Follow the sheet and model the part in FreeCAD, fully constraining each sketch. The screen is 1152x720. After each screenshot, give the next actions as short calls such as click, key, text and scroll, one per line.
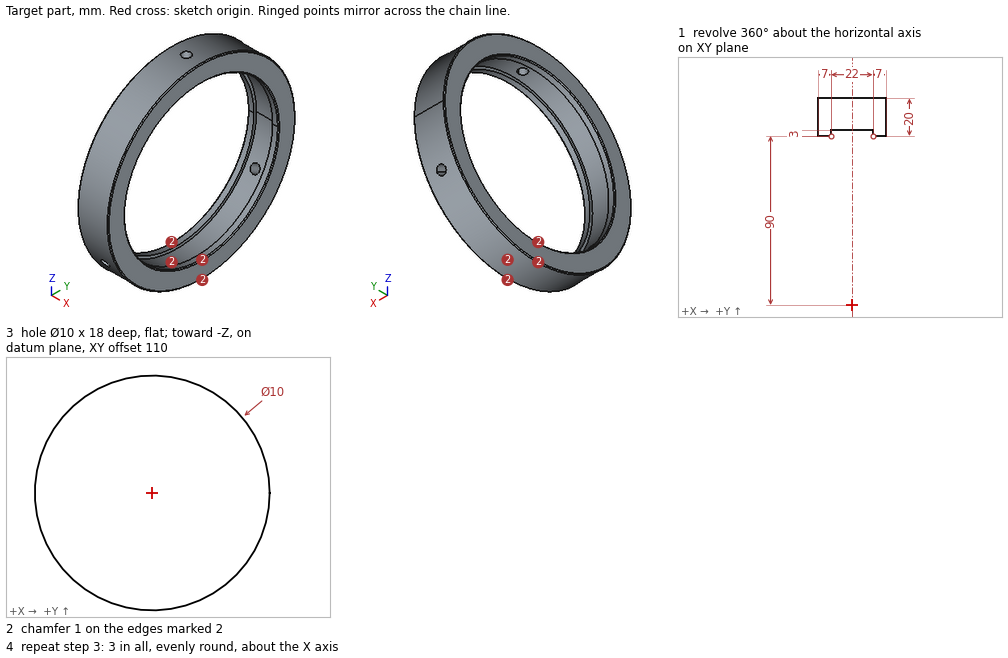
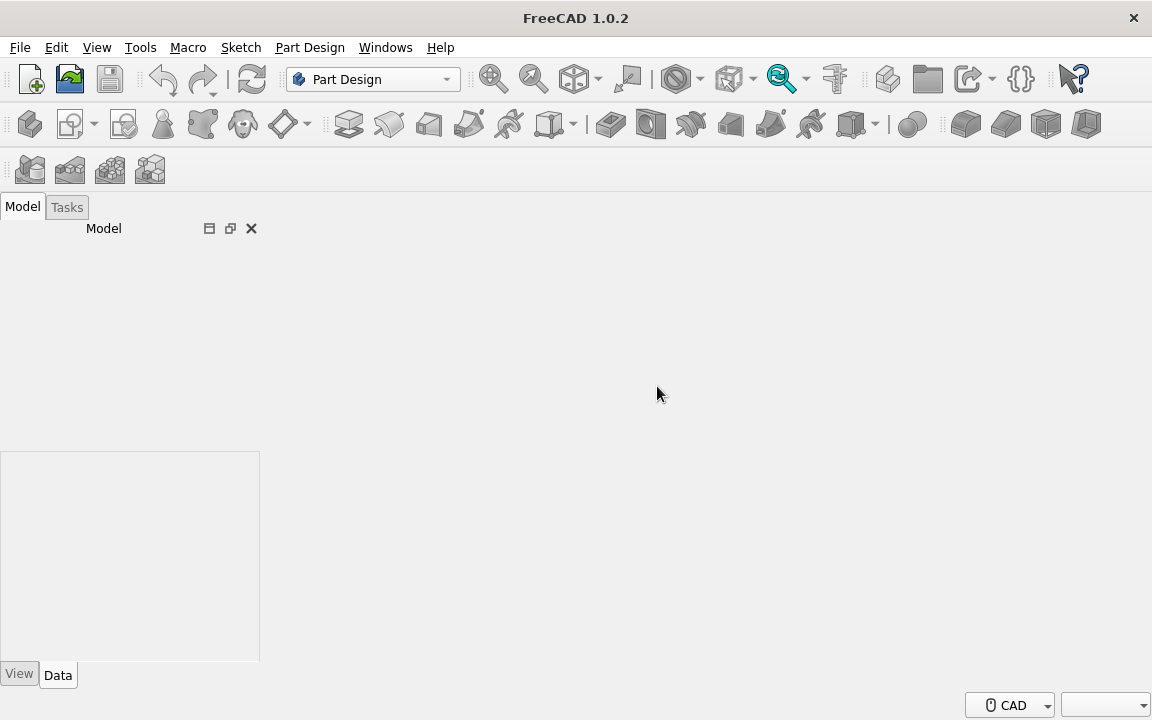
click(30, 80)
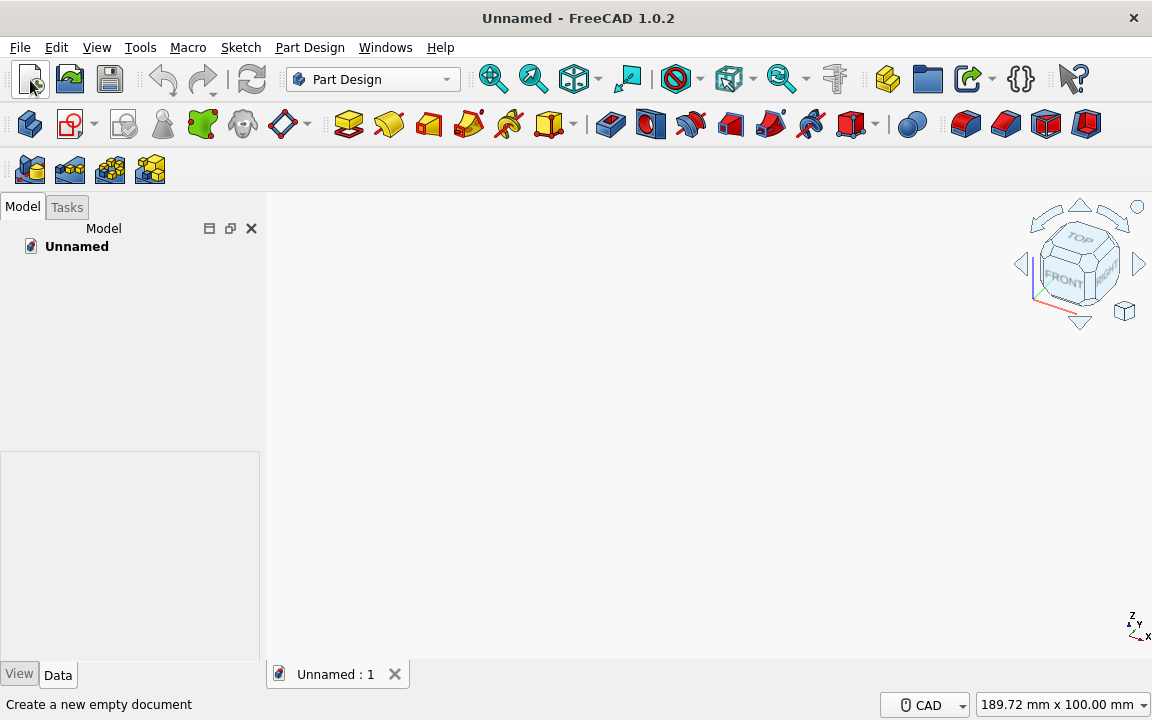
click(70, 124)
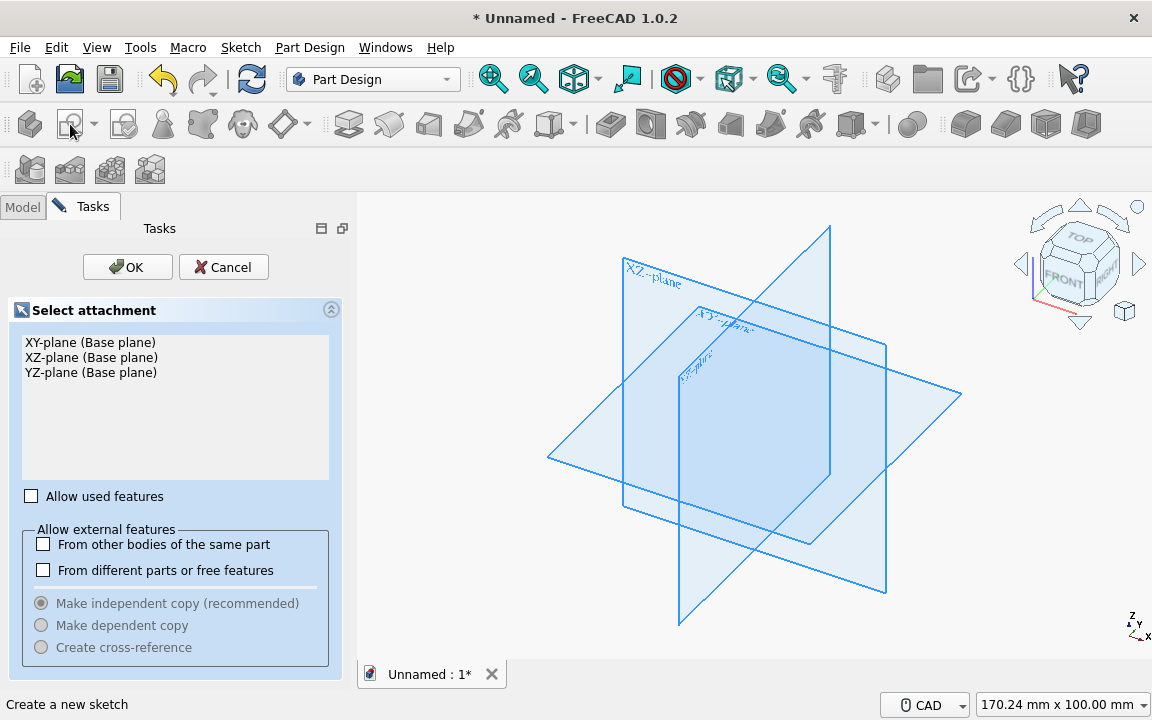
click(82, 342)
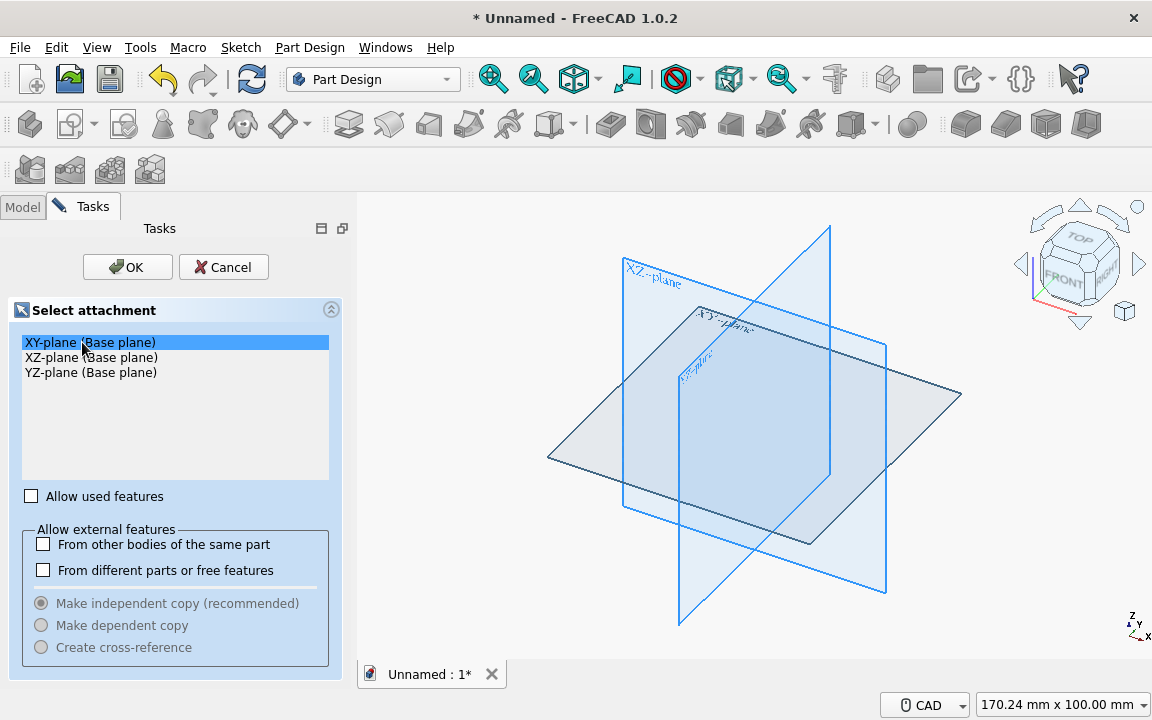
click(128, 267)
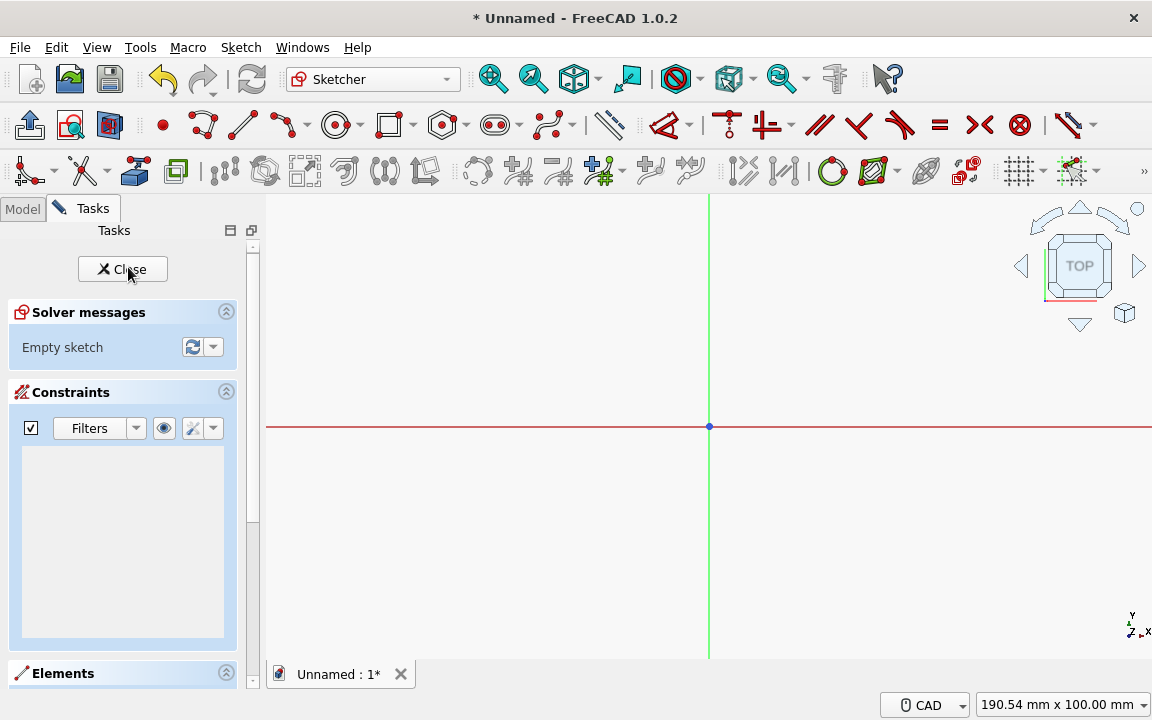
scroll(640, 426, down, 5)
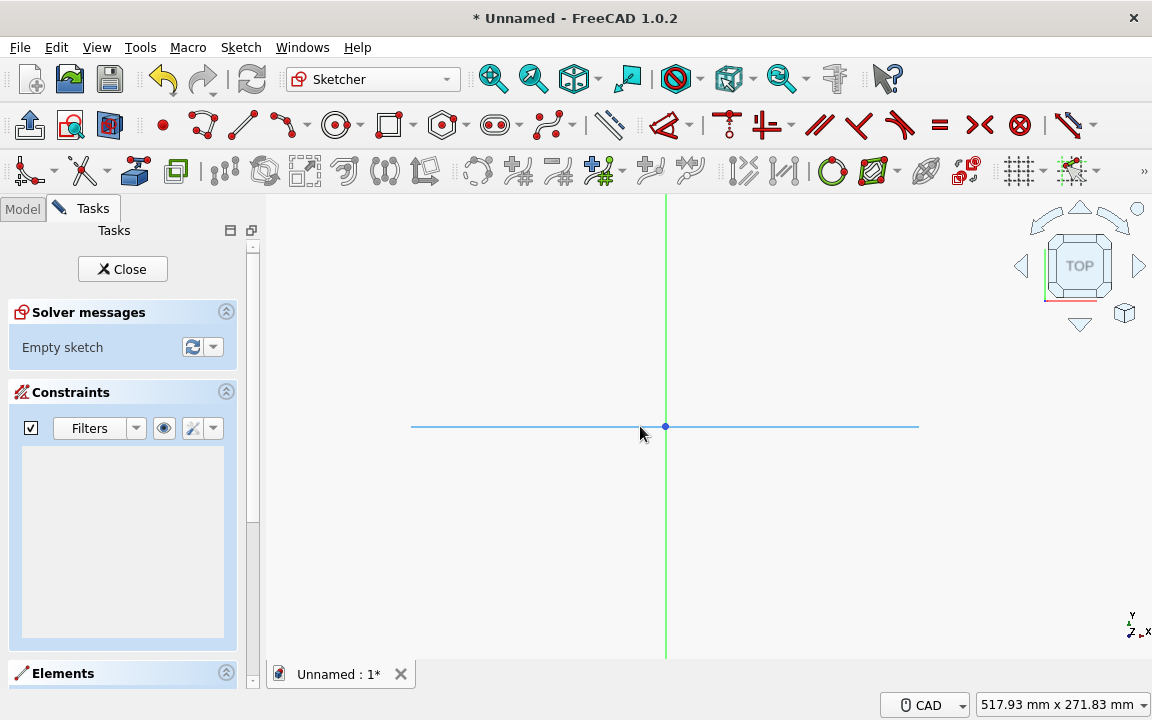
scroll(670, 229, up, 10)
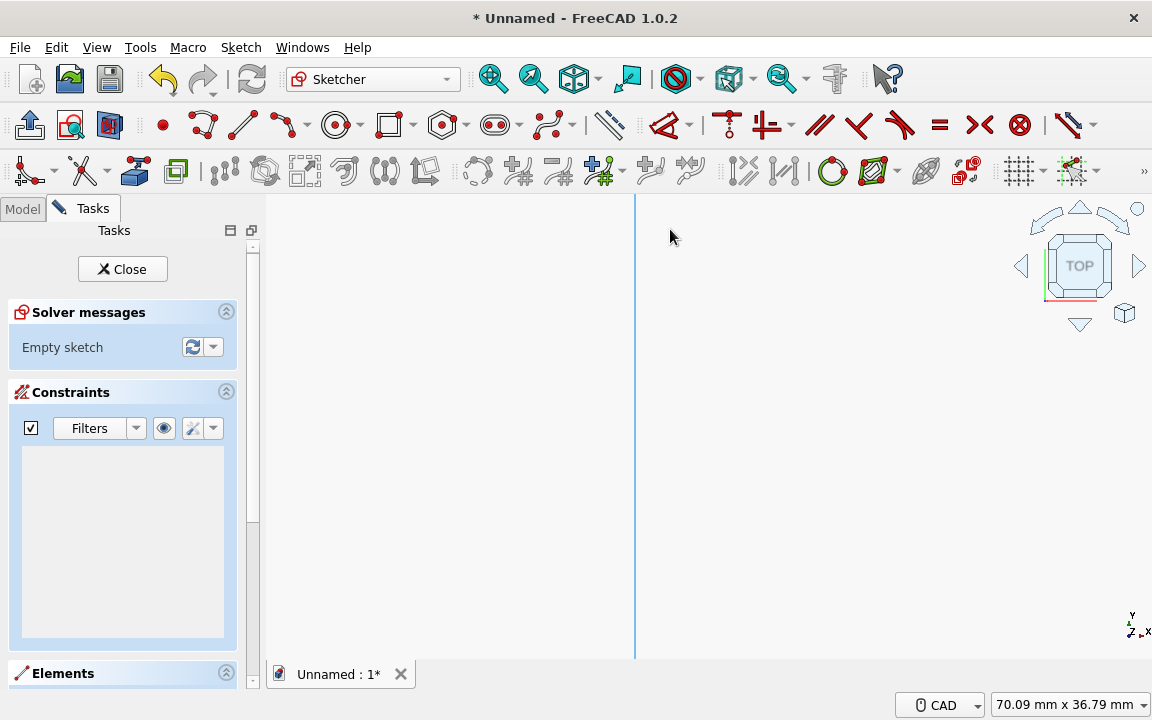
click(204, 126)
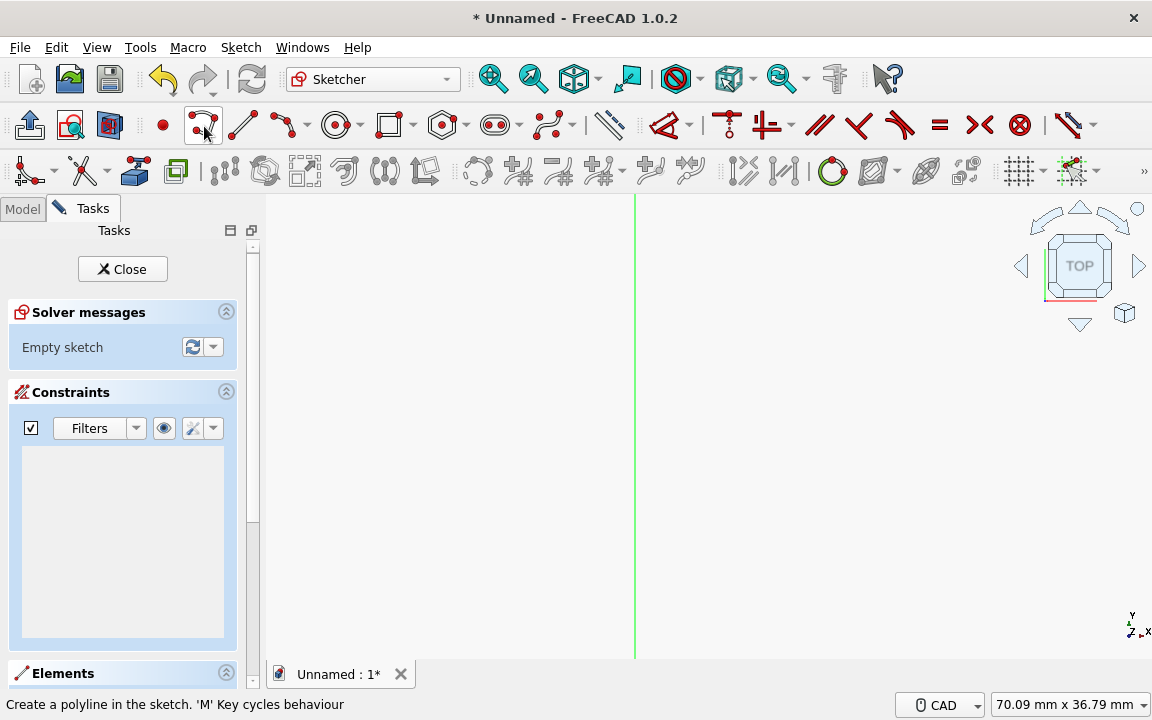
click(496, 550)
click(496, 512)
click(774, 512)
click(774, 550)
click(862, 550)
click(862, 297)
click(407, 297)
click(407, 550)
click(496, 551)
key(Escape)
key(Escape)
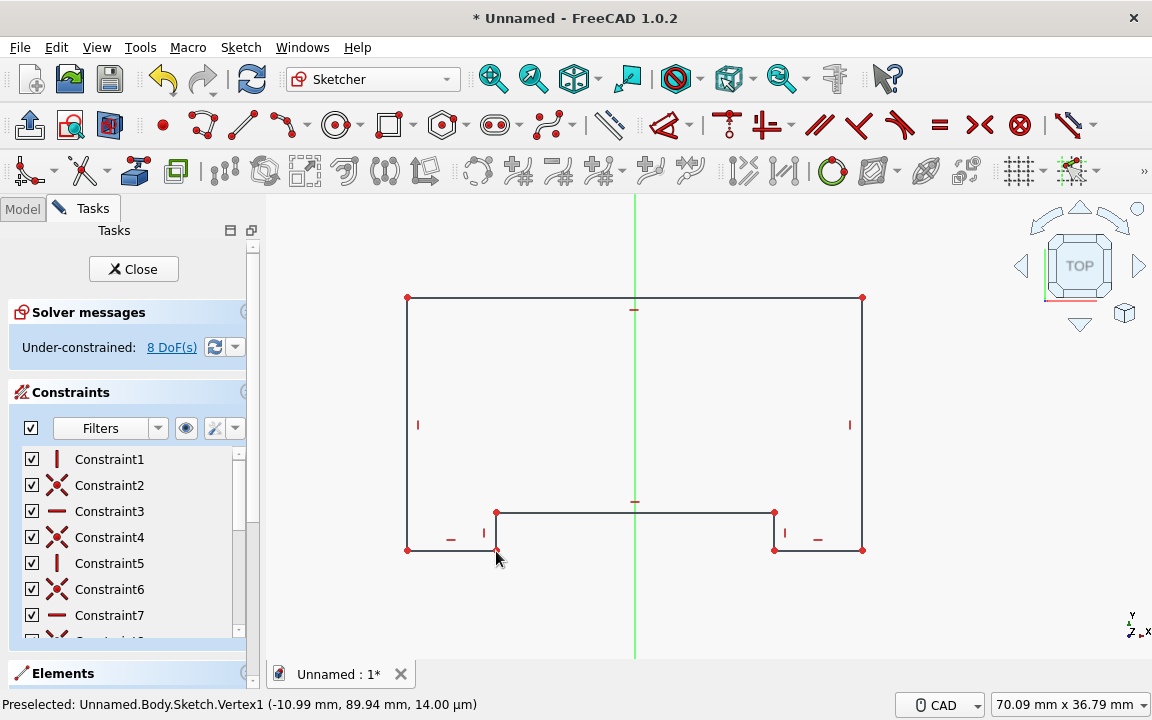
click(496, 551)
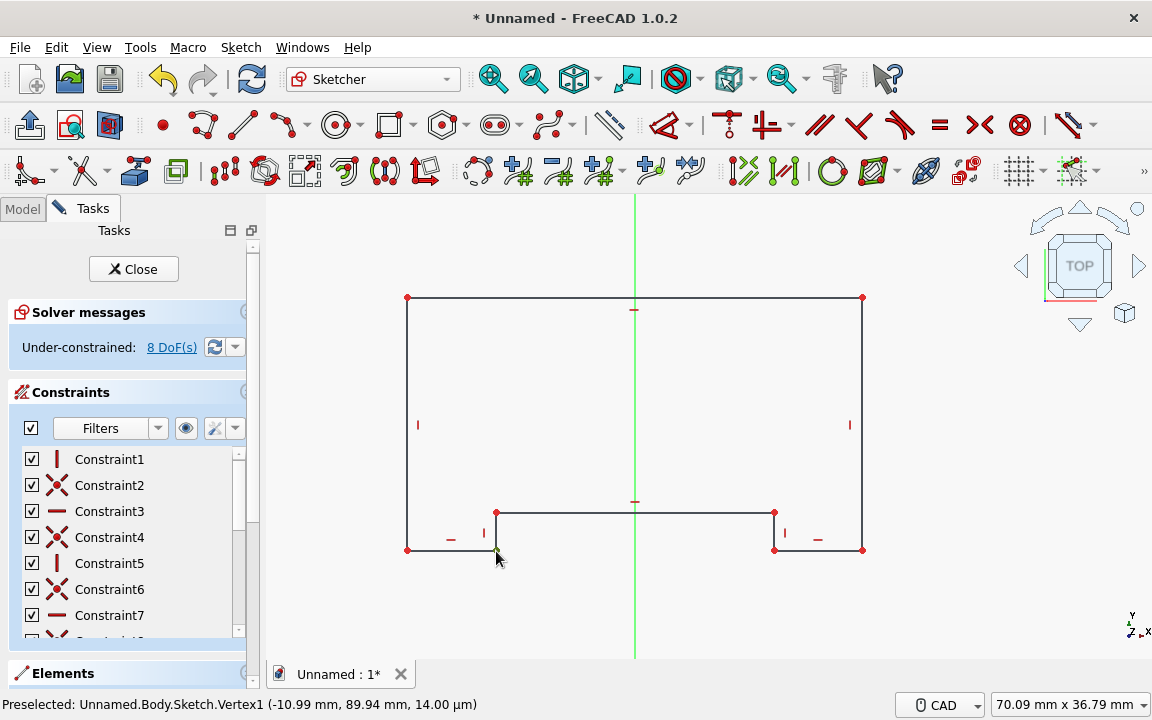
click(774, 551)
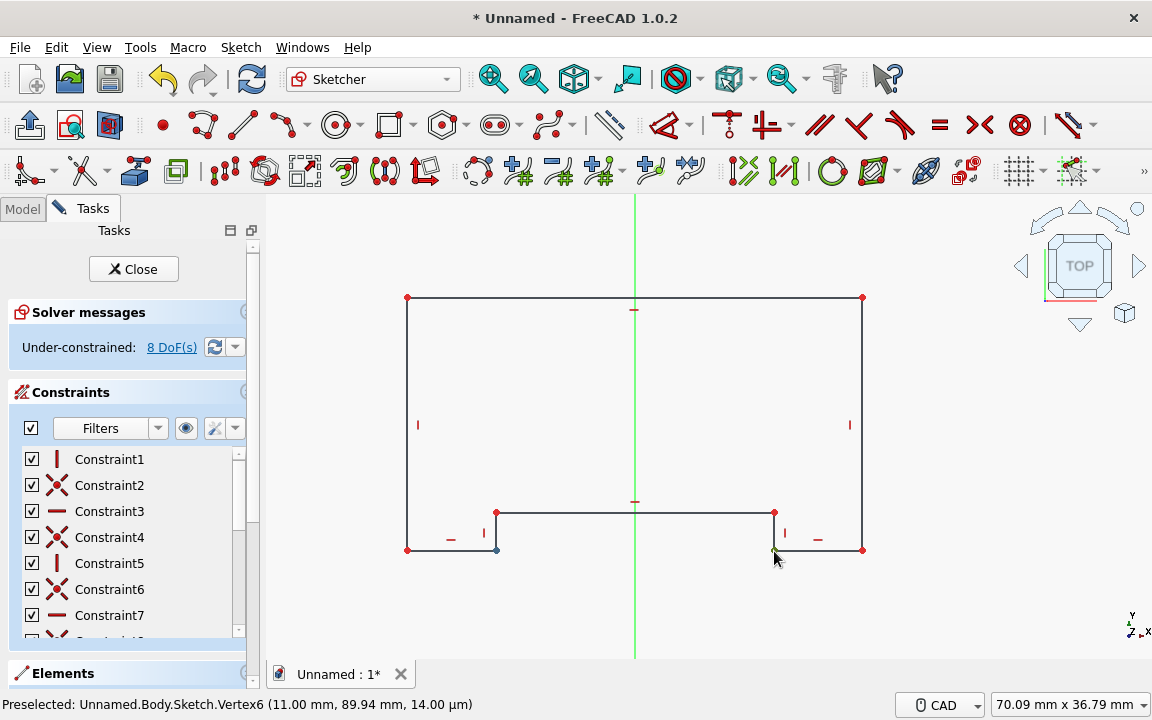
click(635, 602)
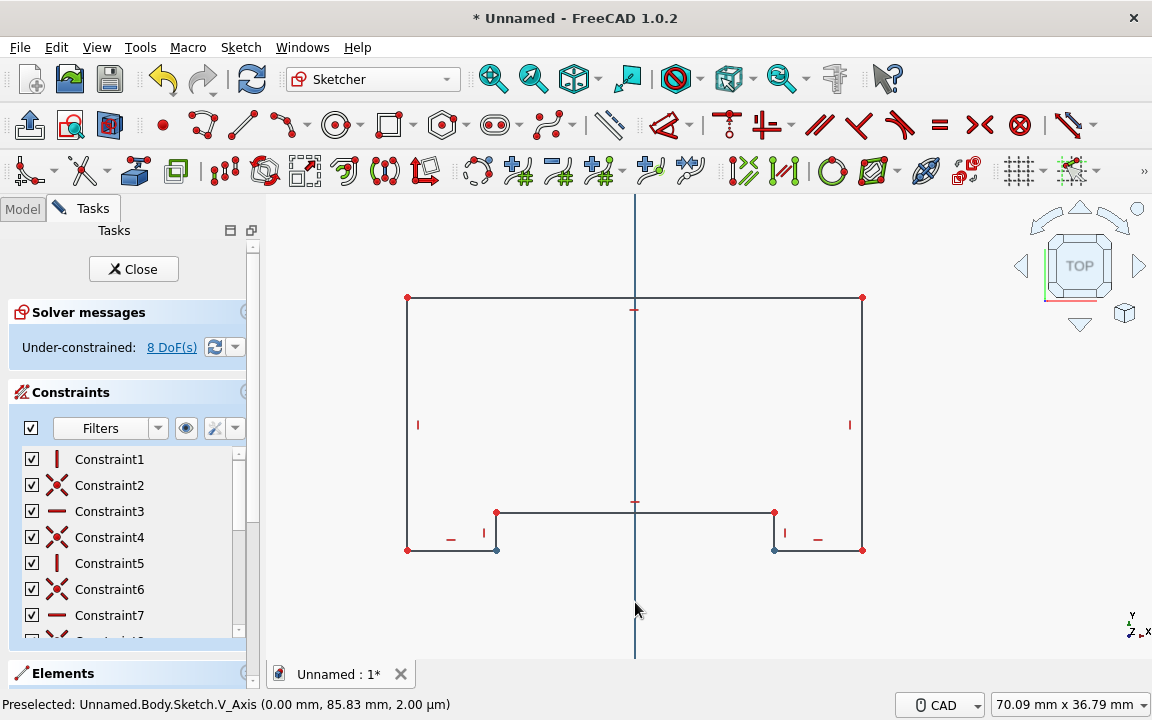
click(980, 126)